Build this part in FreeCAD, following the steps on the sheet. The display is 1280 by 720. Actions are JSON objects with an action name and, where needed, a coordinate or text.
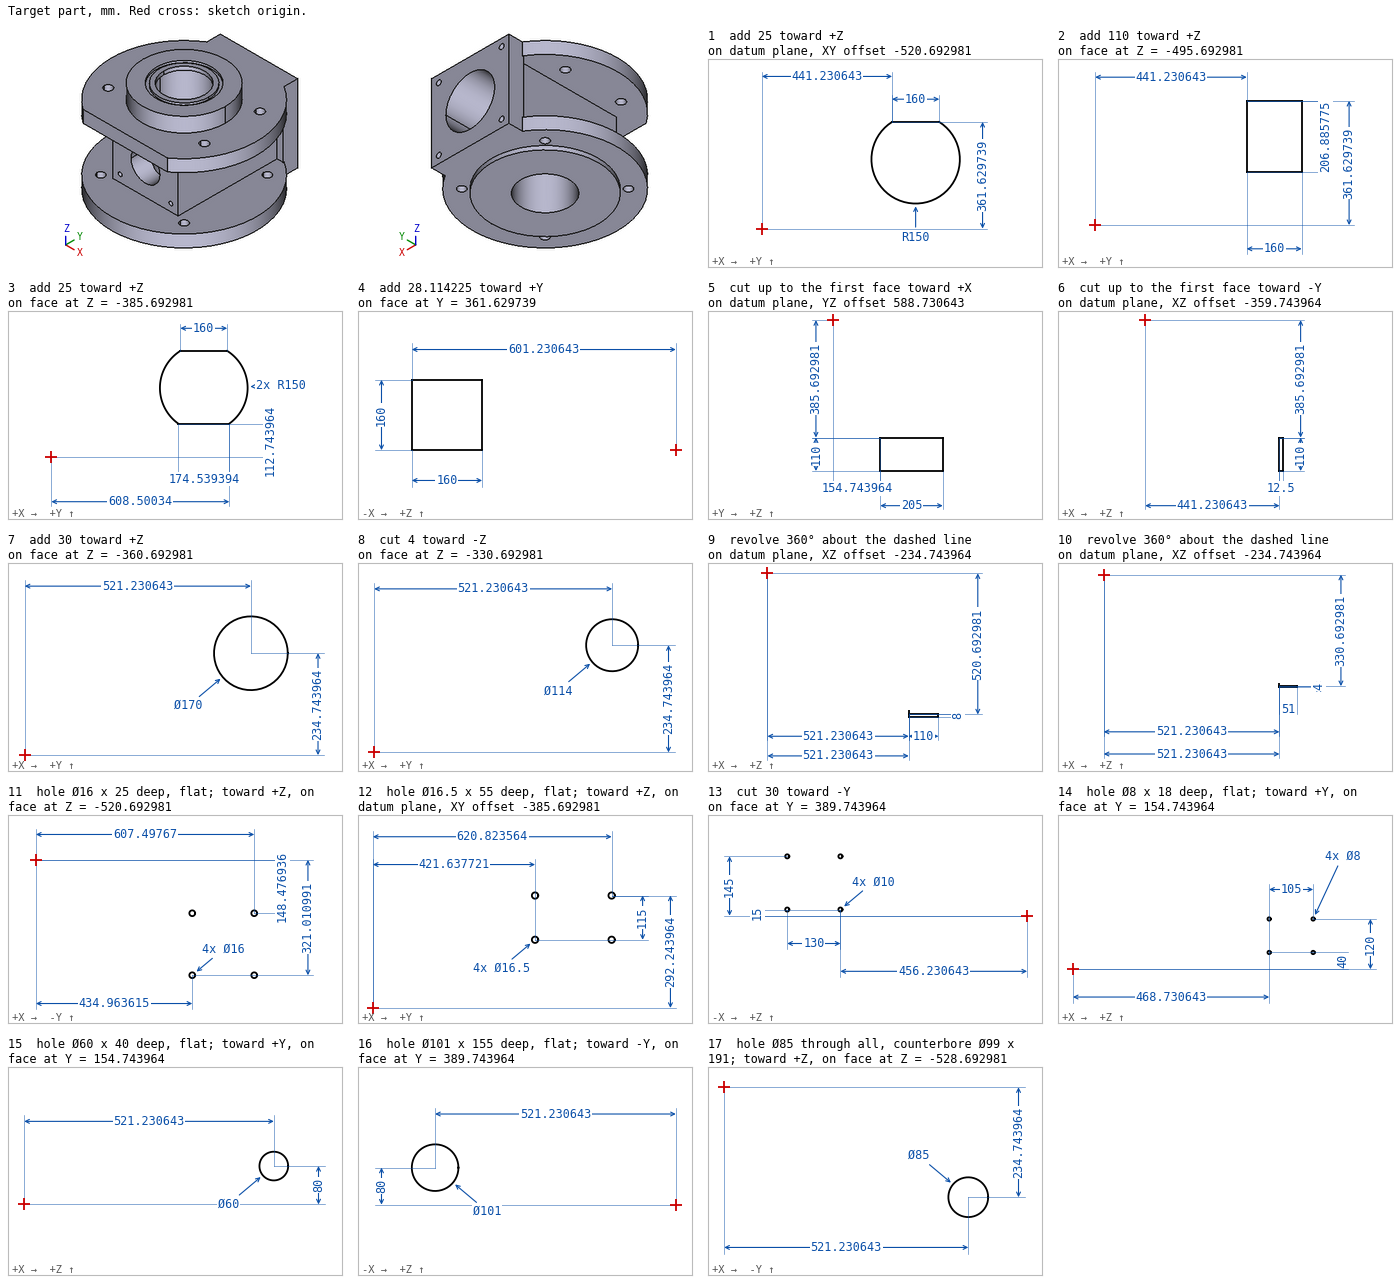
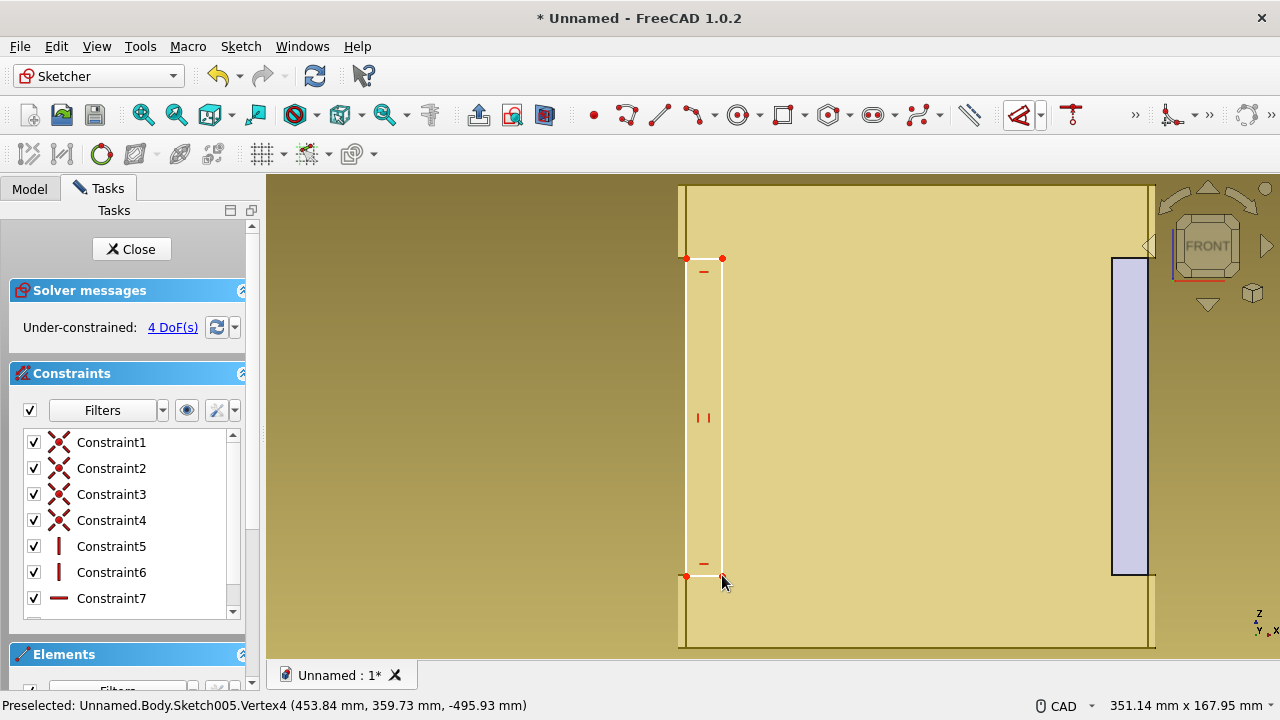
{"action": "left_click", "coordinate": [686, 354]}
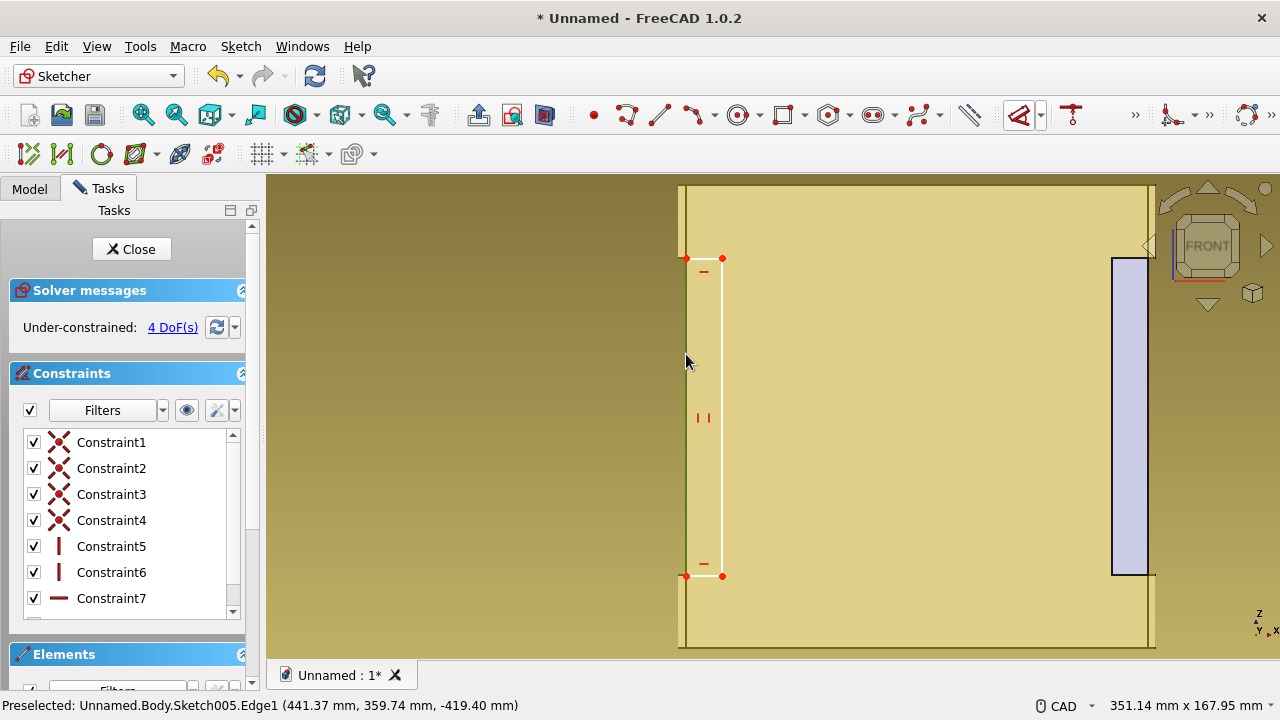
{"action": "left_click", "coordinate": [1040, 116]}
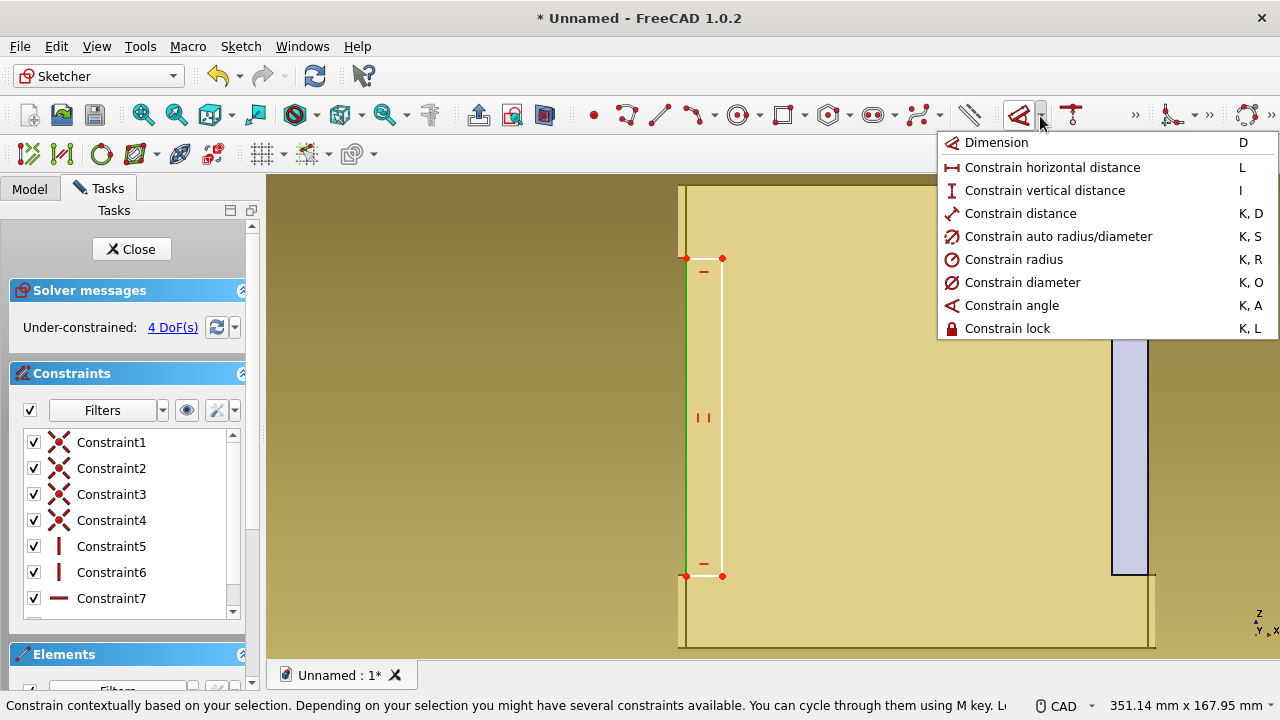
{"action": "left_click", "coordinate": [1108, 190]}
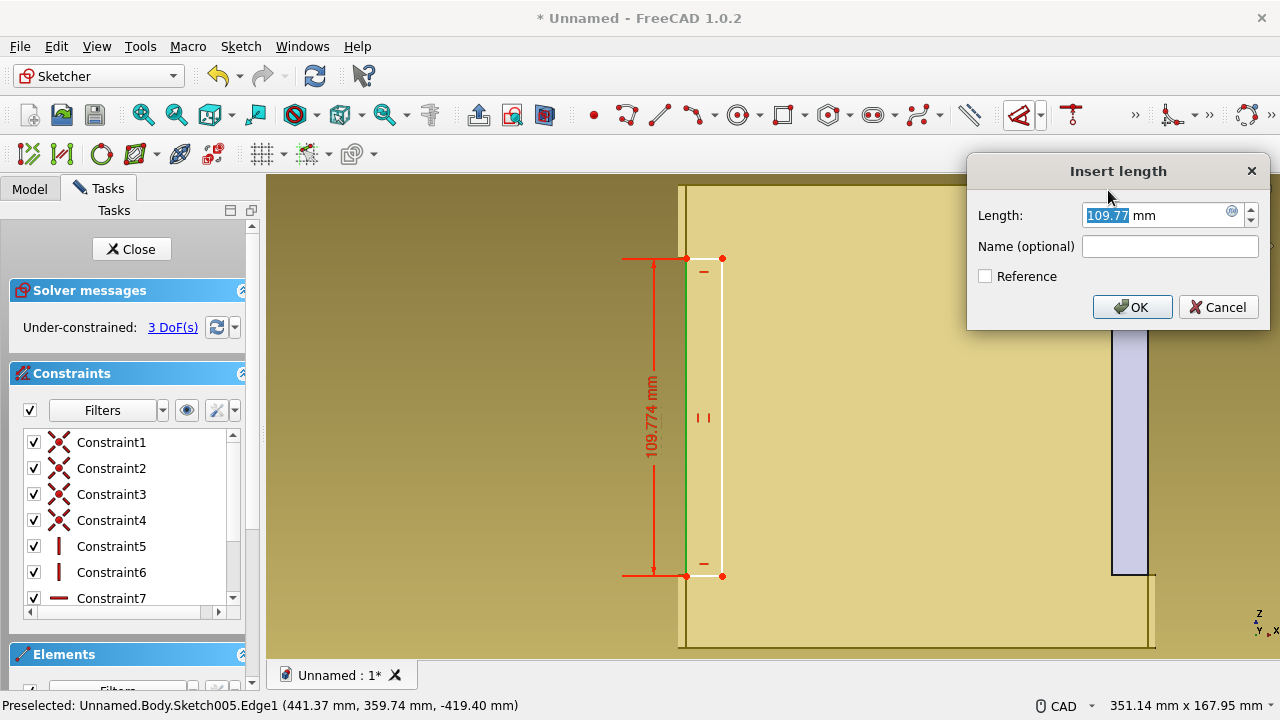
{"action": "type", "text": "110"}
{"action": "key", "text": "Return"}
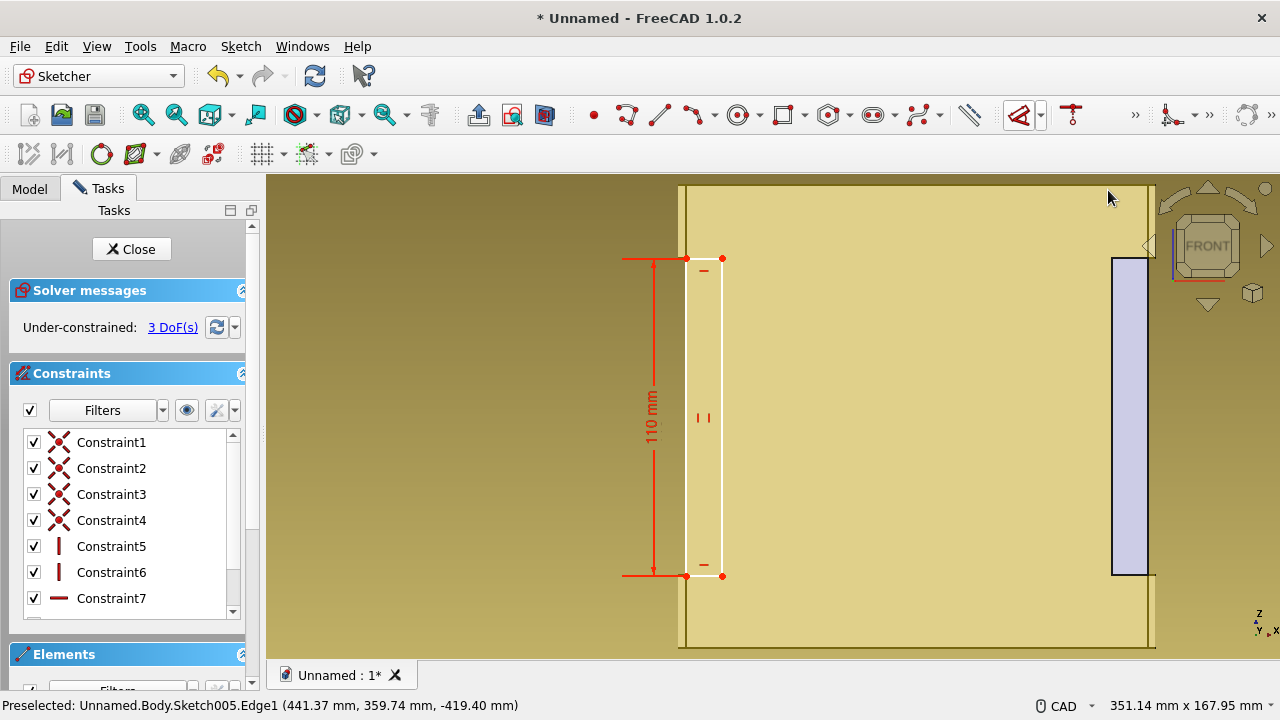
{"action": "scroll", "coordinate": [697, 576], "scroll_direction": "up", "scroll_amount": 2}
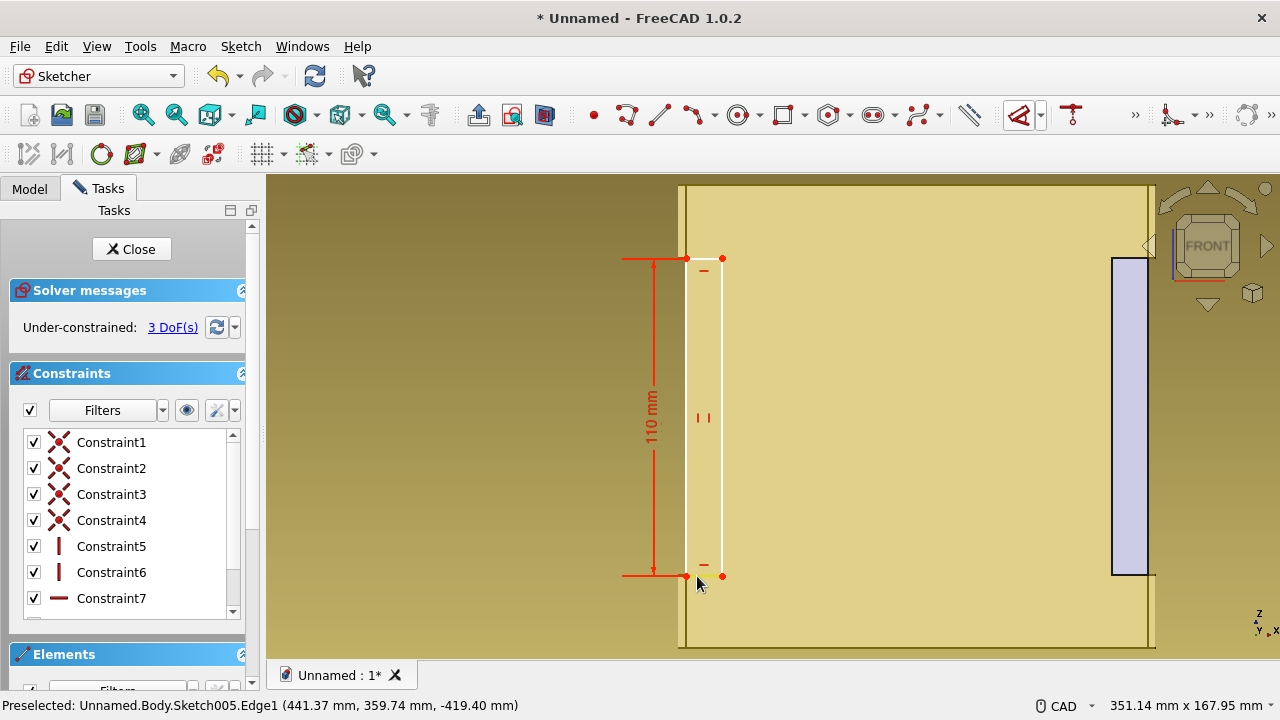
{"action": "left_click", "coordinate": [696, 576]}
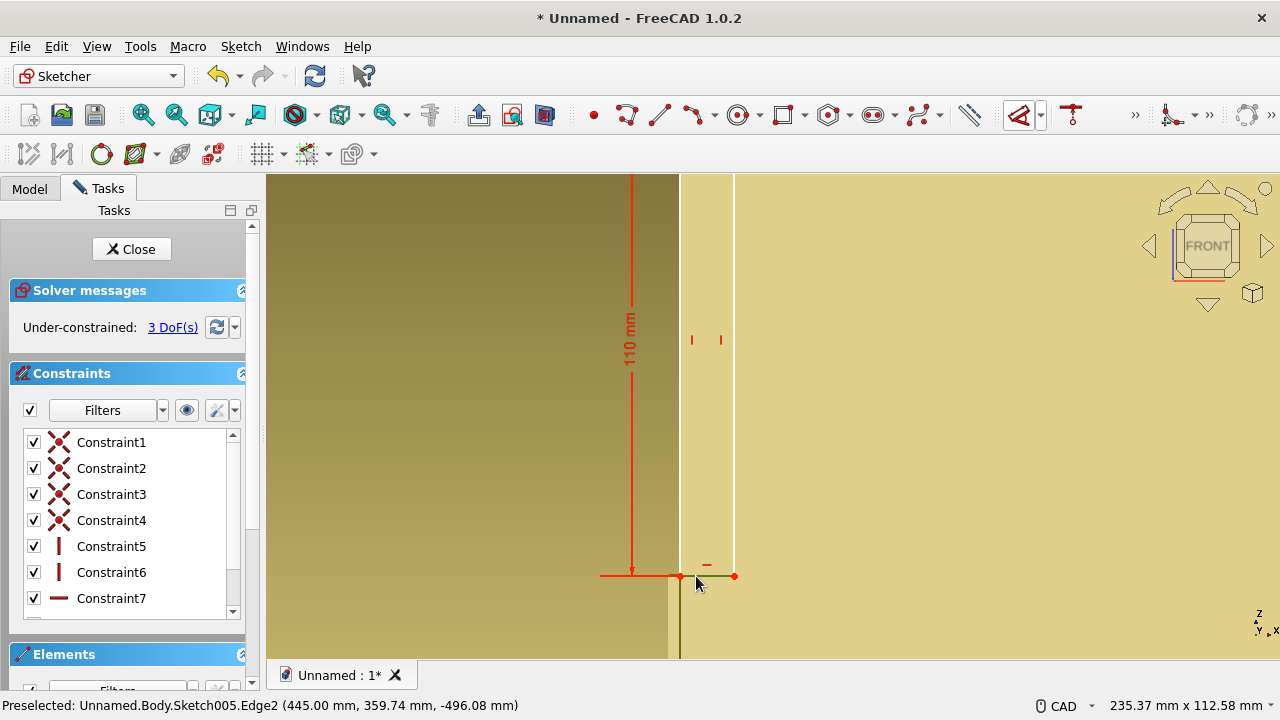
{"action": "left_click", "coordinate": [1040, 116]}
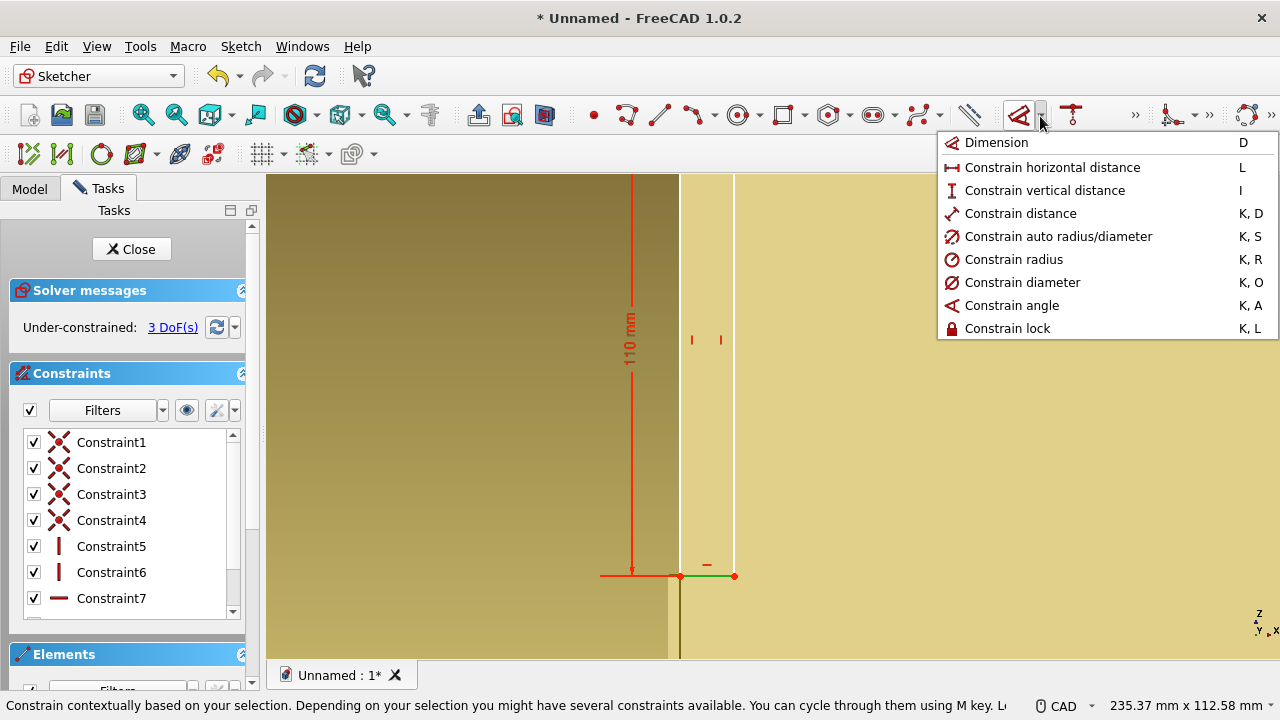
{"action": "left_click", "coordinate": [1108, 168]}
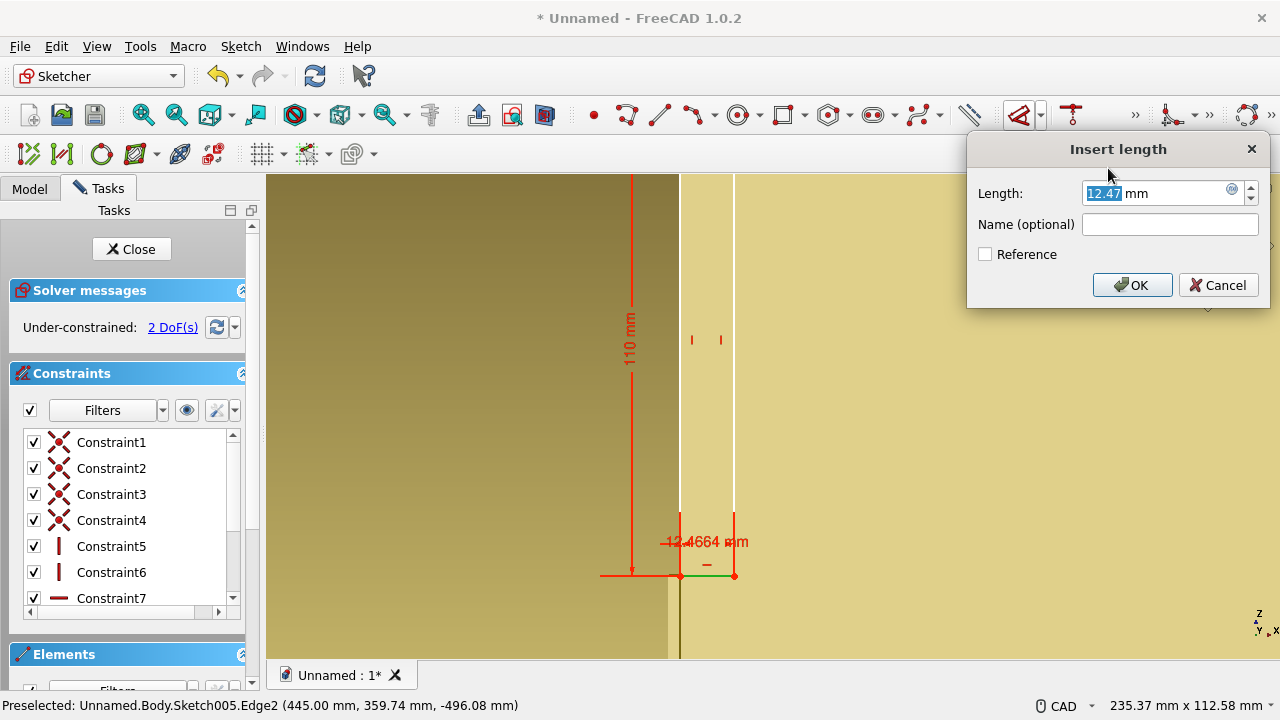
{"action": "type", "text": "12.5"}
{"action": "key", "text": "Return"}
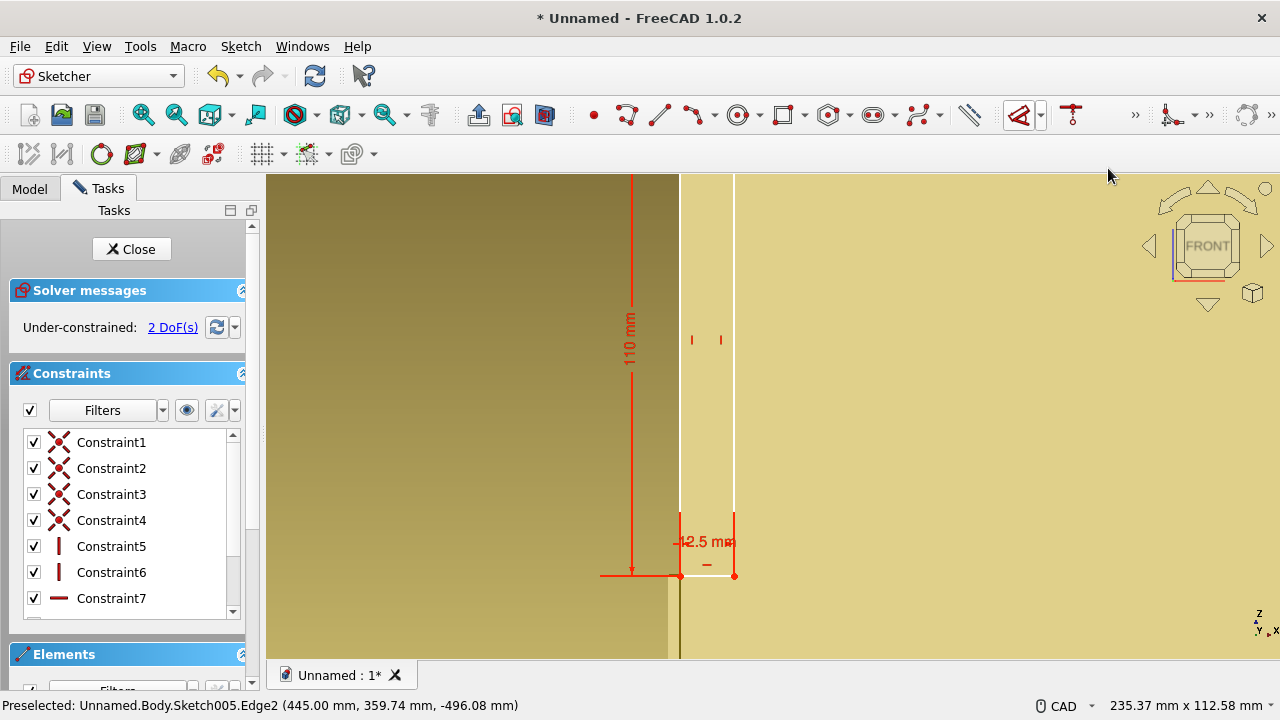
{"action": "scroll", "coordinate": [700, 577], "scroll_direction": "down", "scroll_amount": 2}